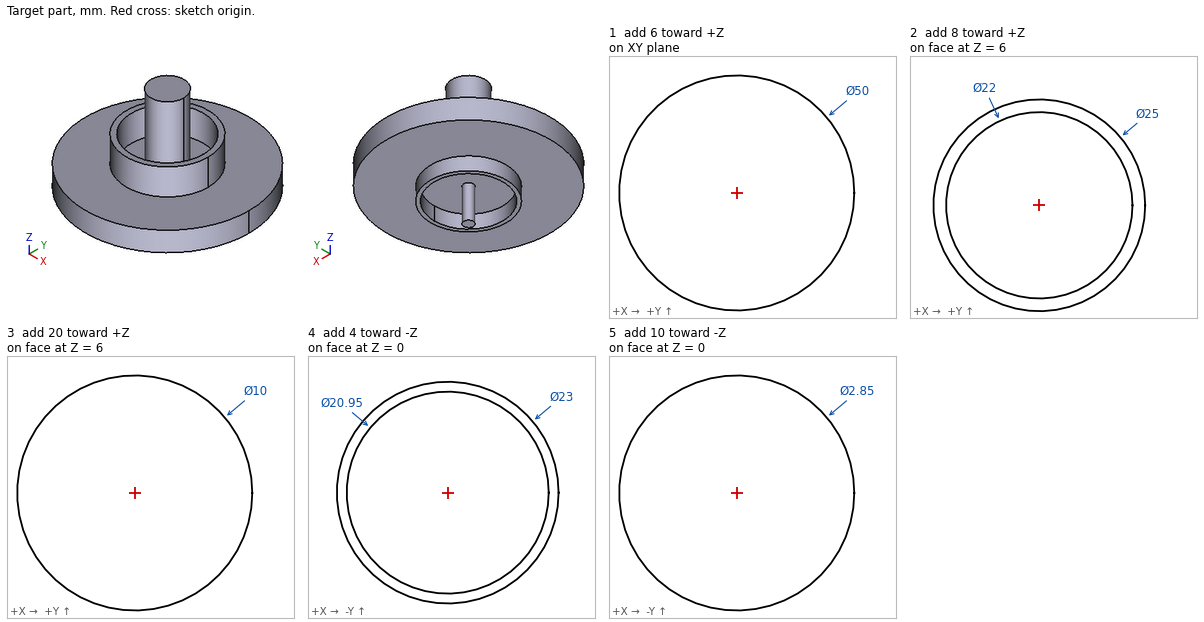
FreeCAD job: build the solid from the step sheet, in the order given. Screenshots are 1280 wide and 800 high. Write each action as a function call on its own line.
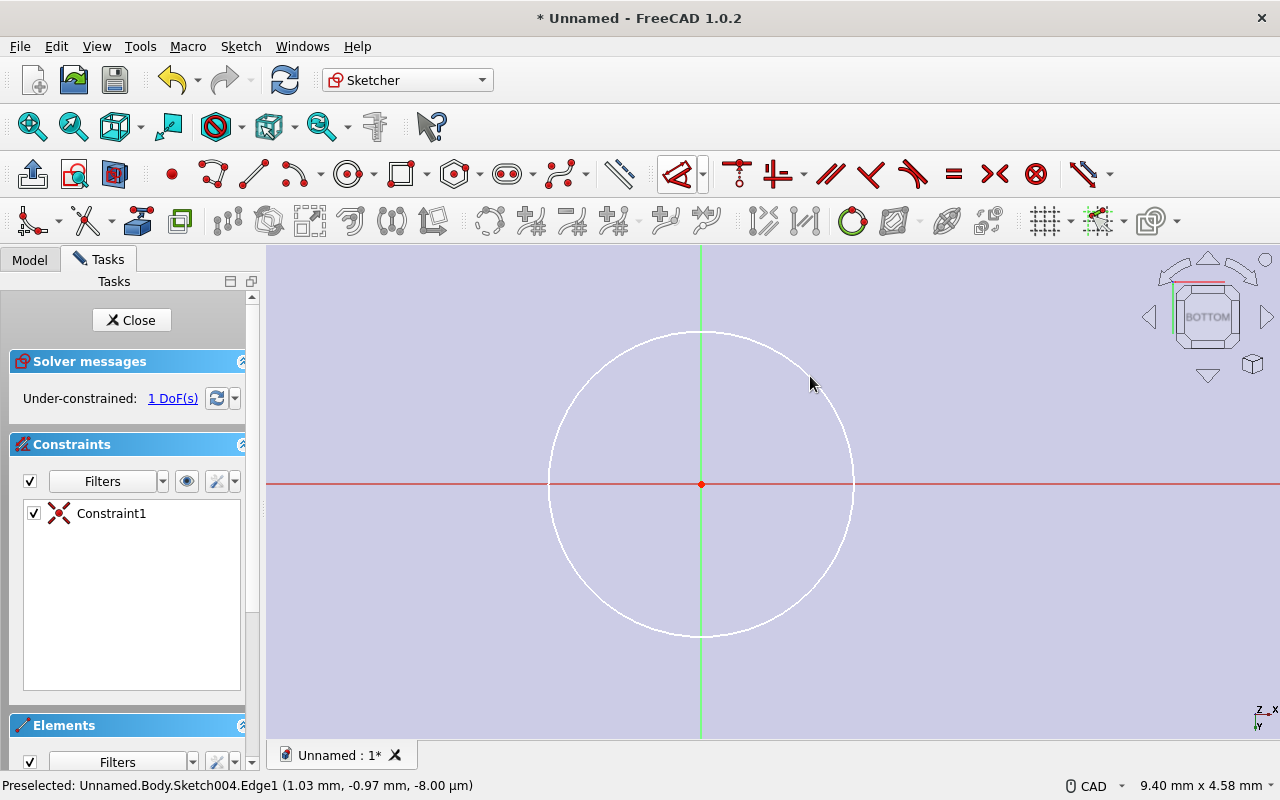
click(809, 376)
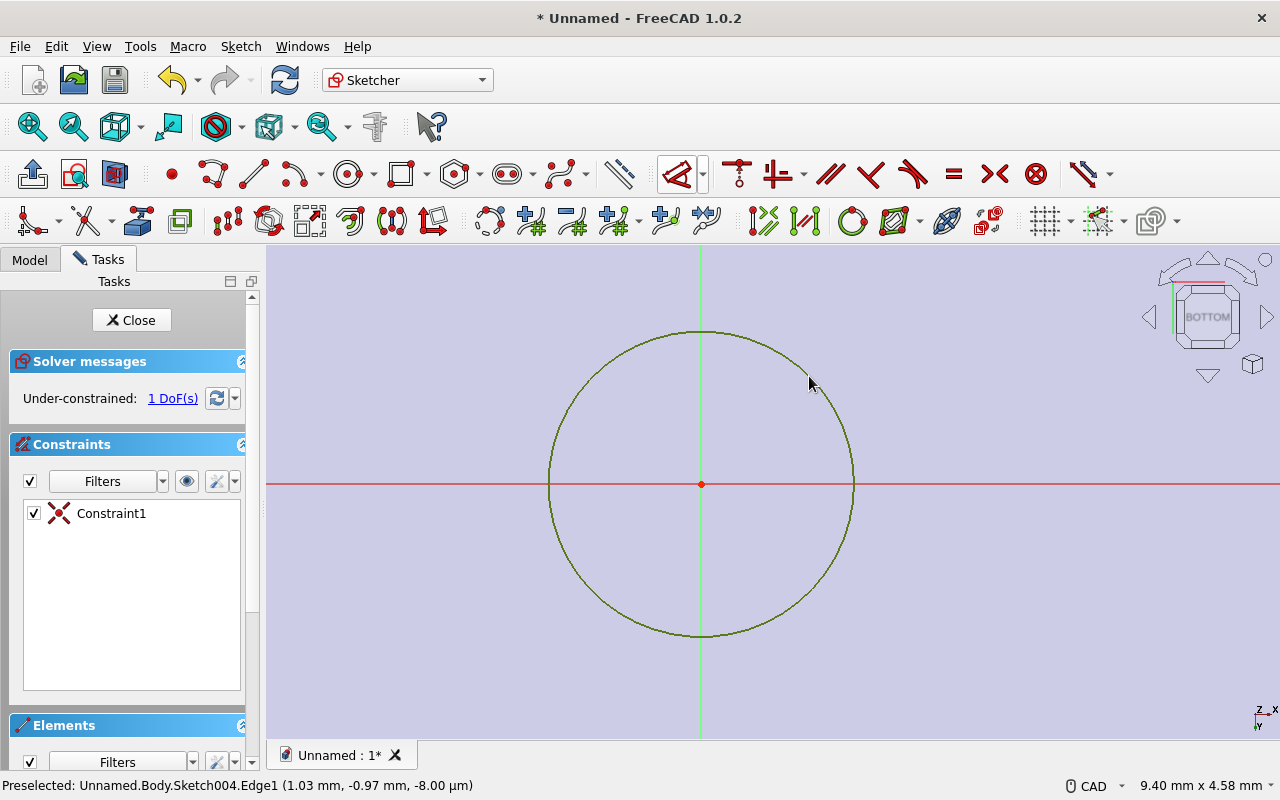
key(k)
key(o)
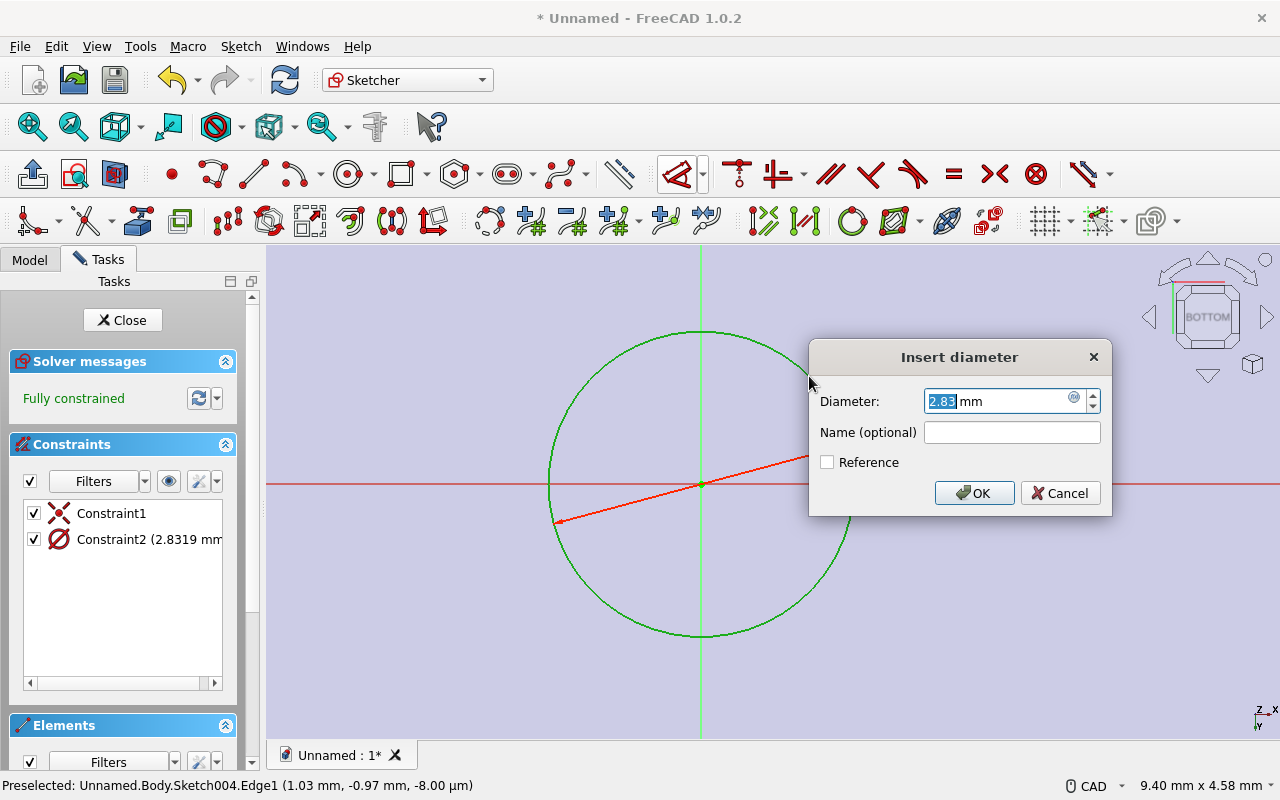
text(2.85)
key(Return)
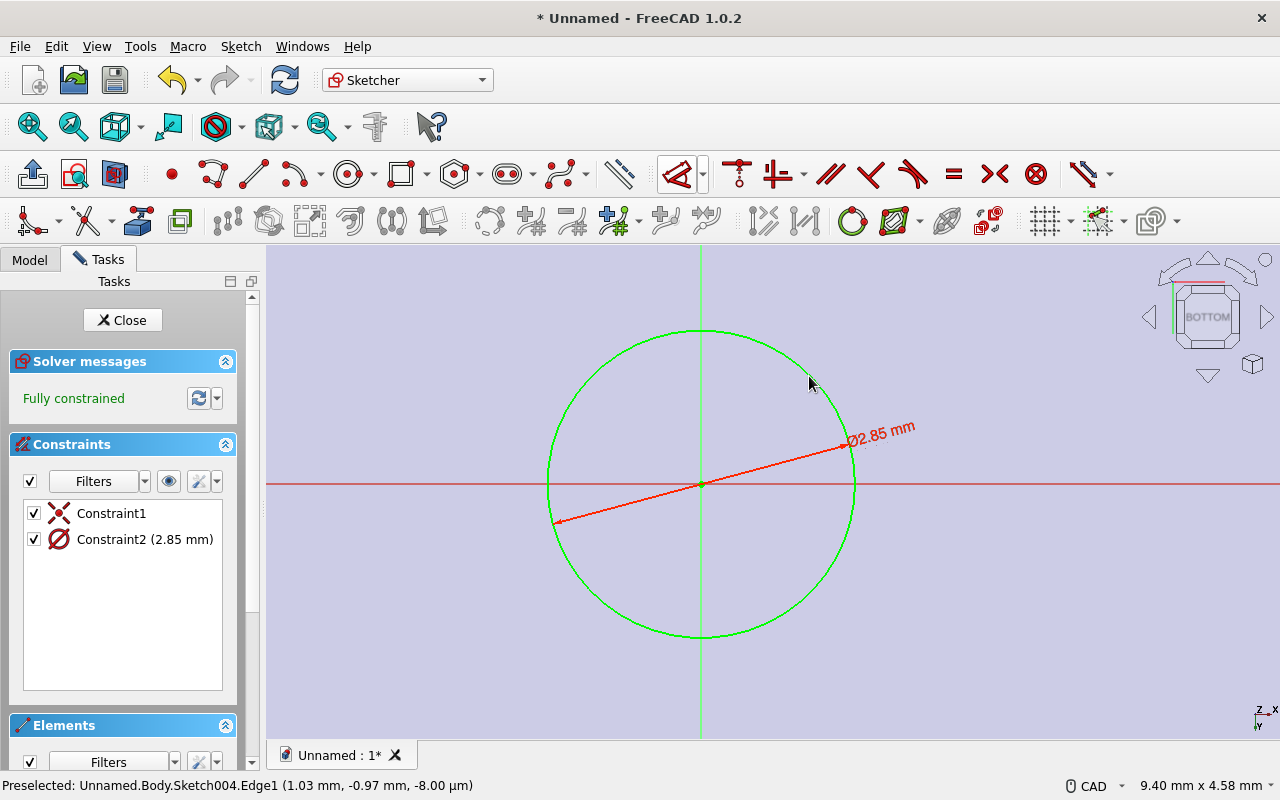
click(123, 320)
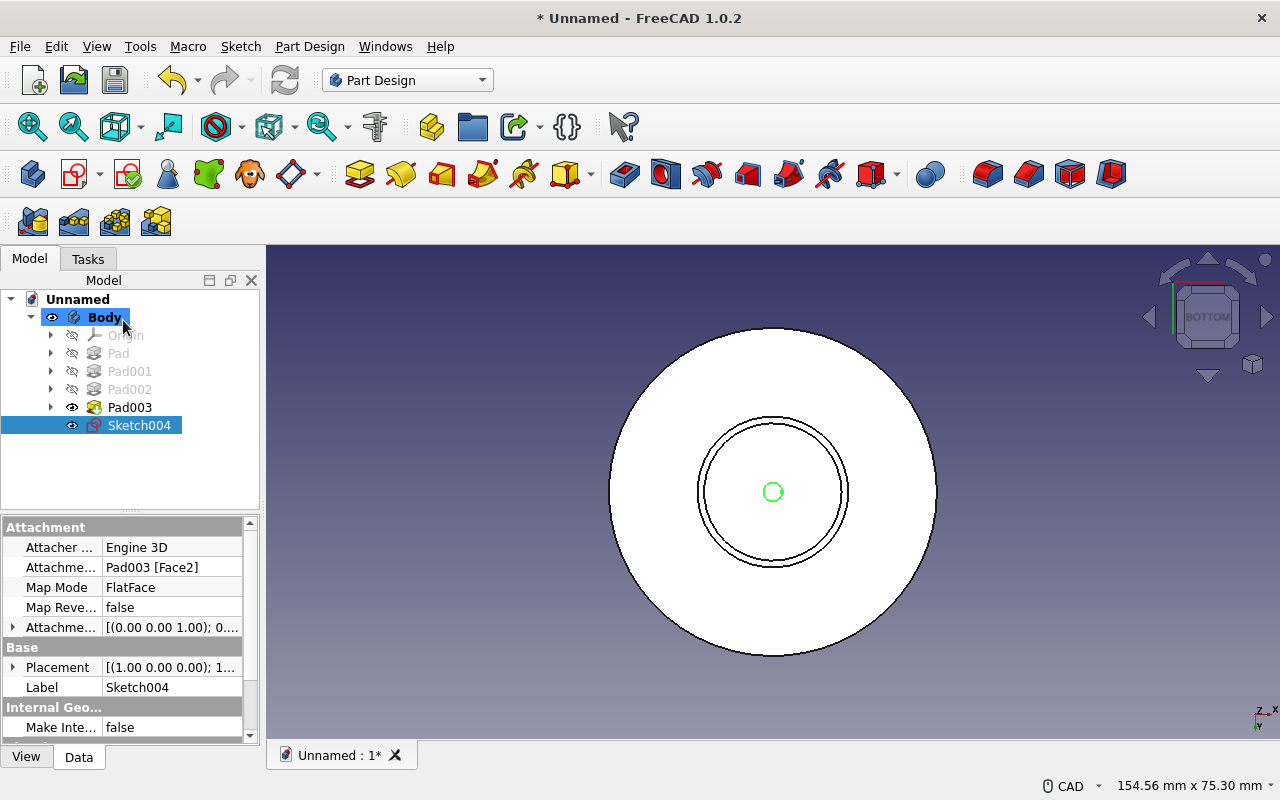
click(360, 174)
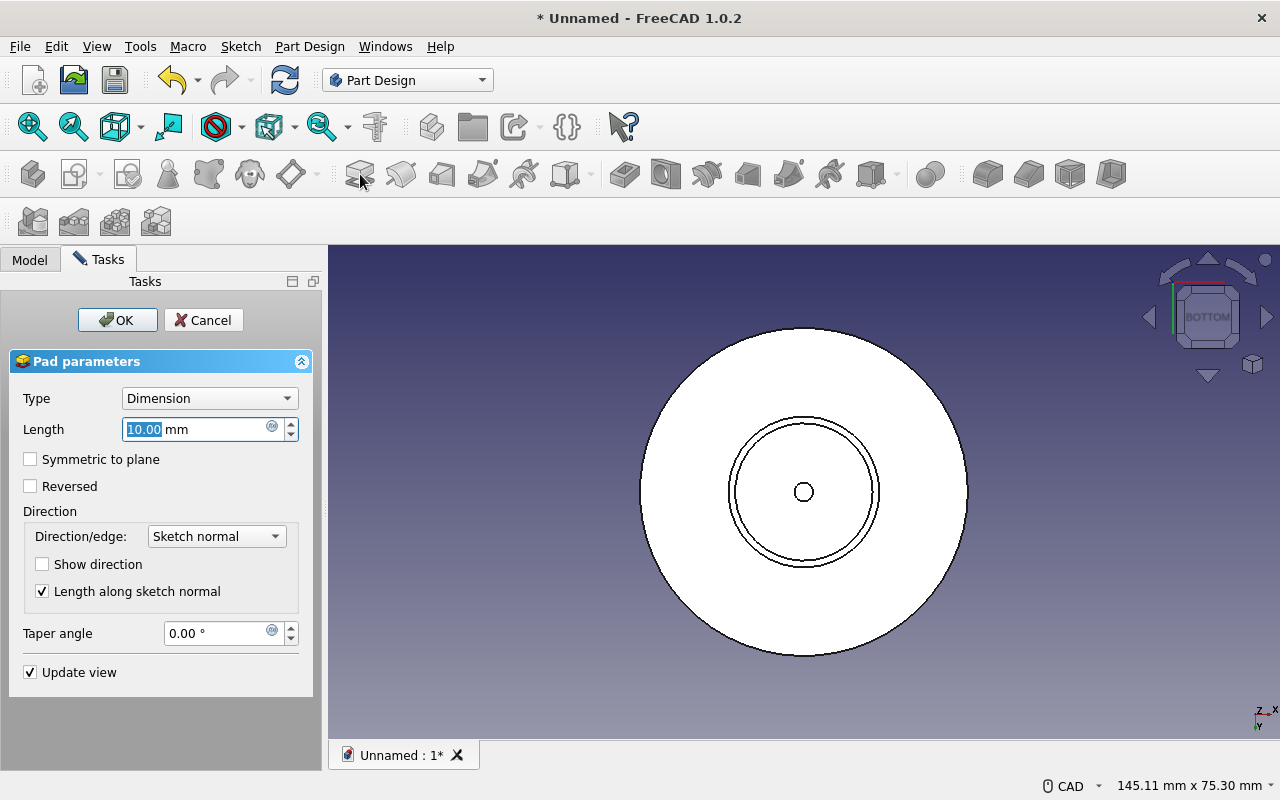
text(10)
key(Tab)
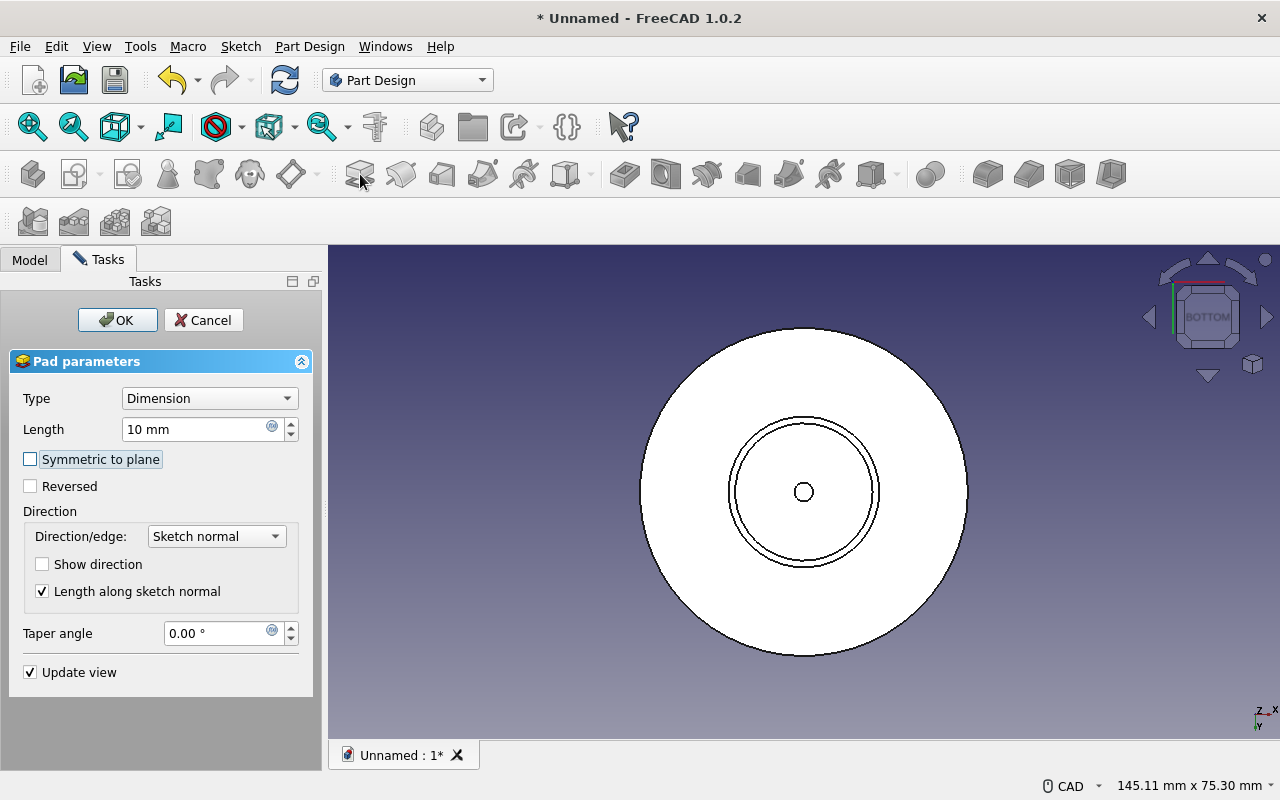
click(118, 320)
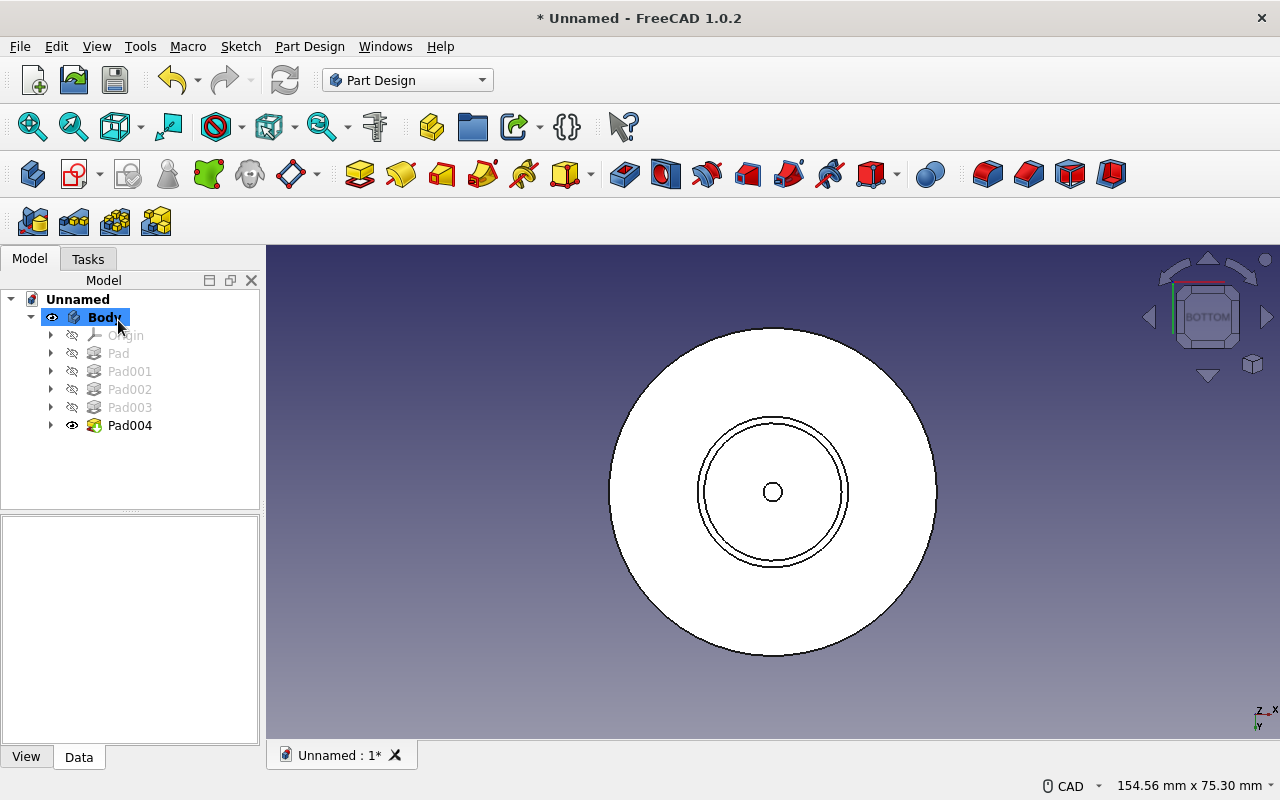
key(0)